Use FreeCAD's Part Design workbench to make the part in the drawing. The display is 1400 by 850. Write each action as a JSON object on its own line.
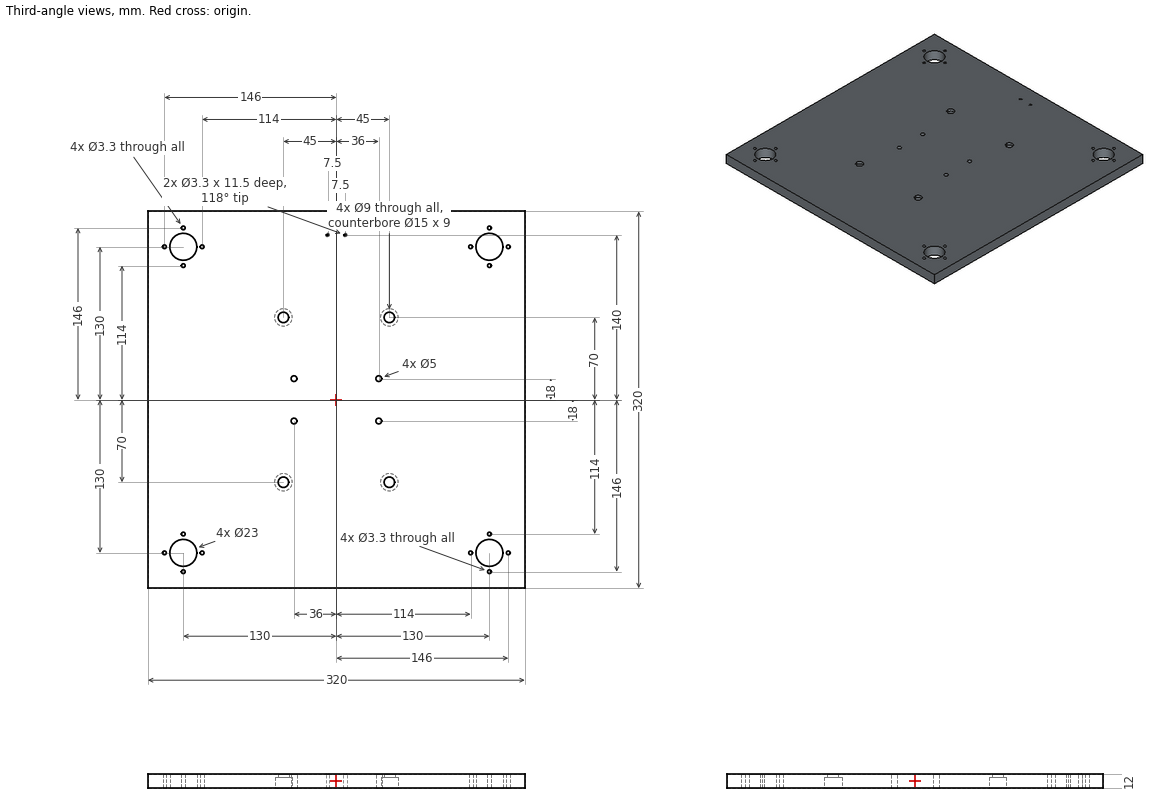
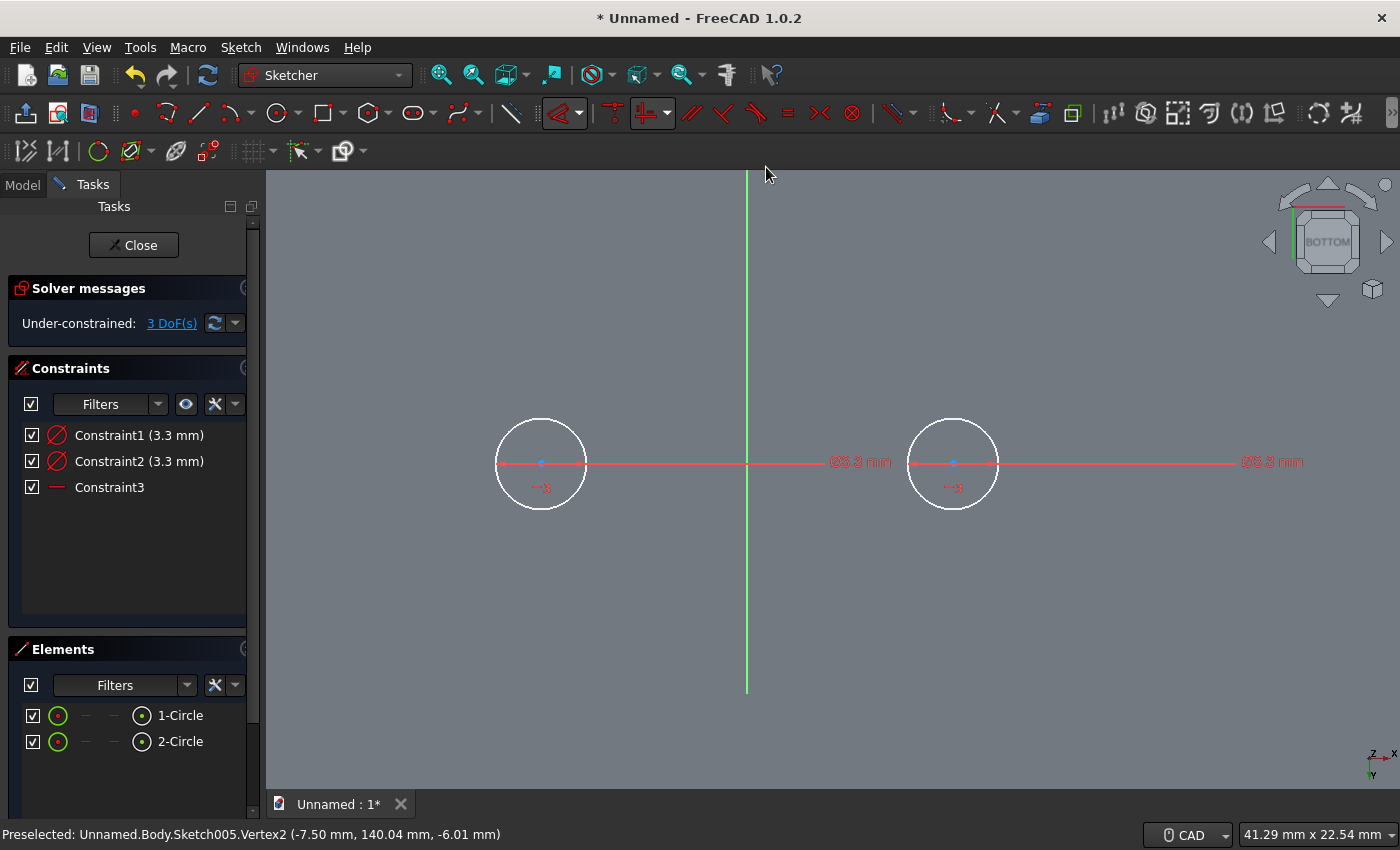
{"action": "left_click", "coordinate": [953, 464]}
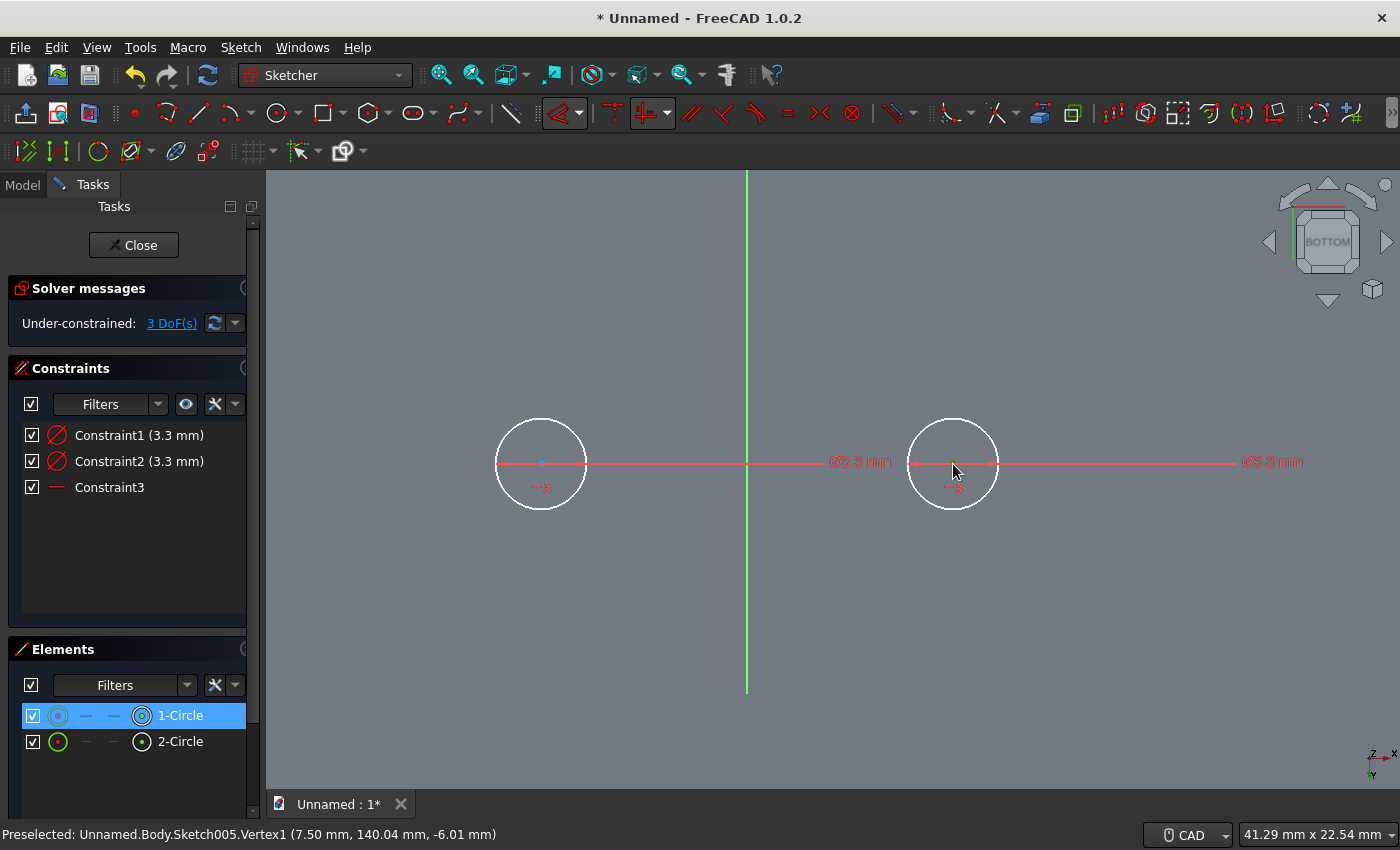
{"action": "key", "text": "l"}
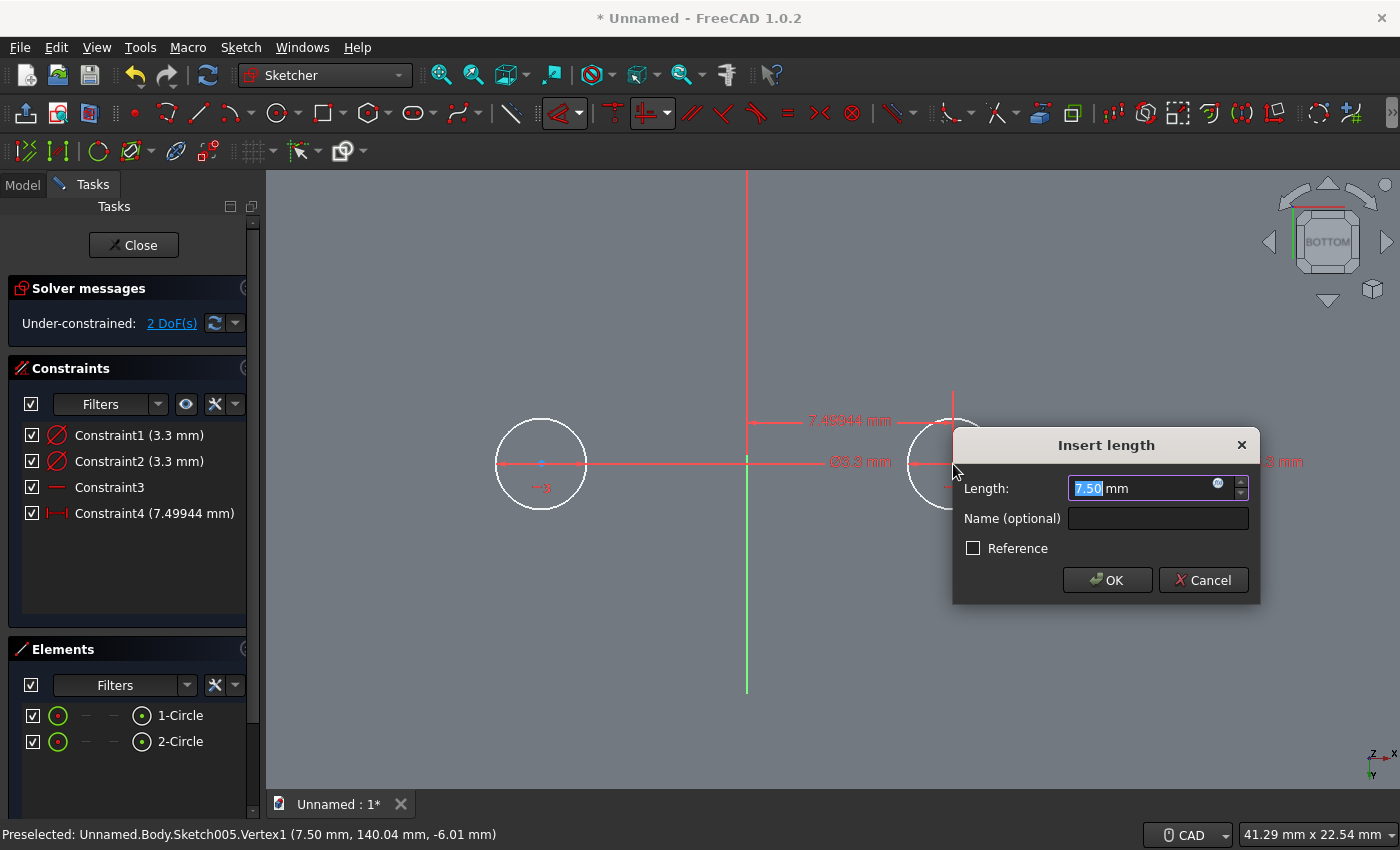
{"action": "type", "text": "7.5"}
{"action": "key", "text": "Return"}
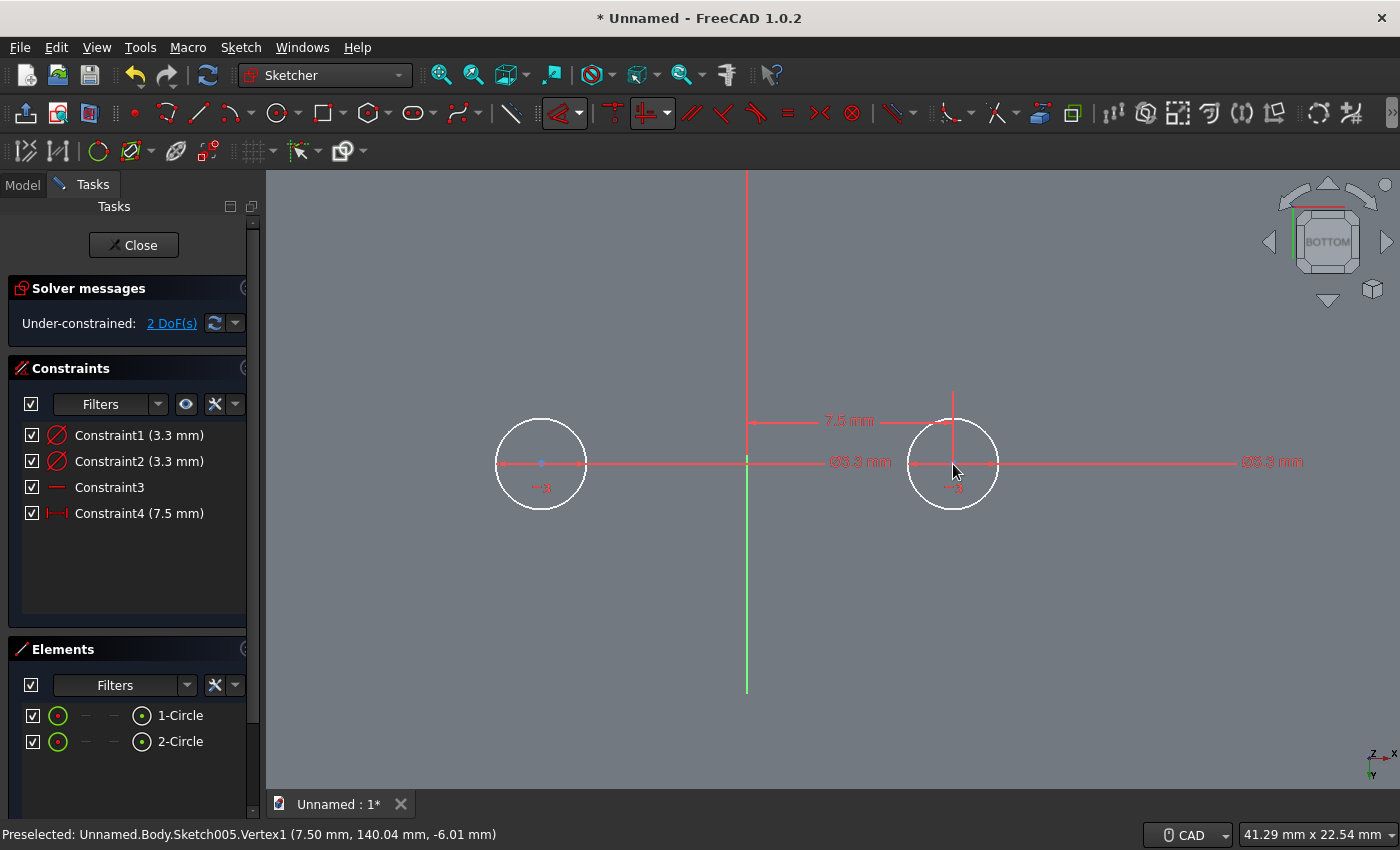
{"action": "left_click", "coordinate": [953, 464]}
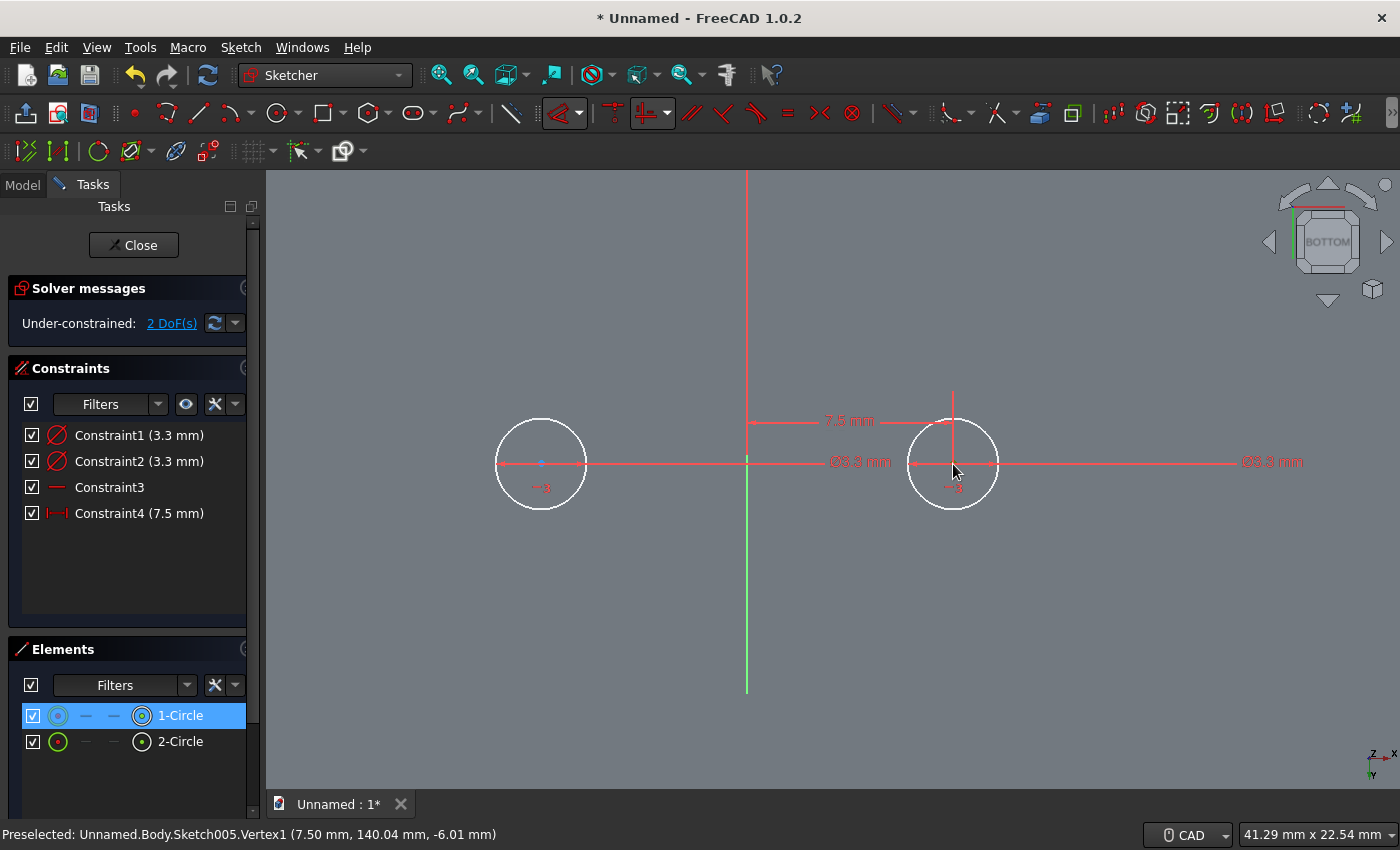
{"action": "left_click", "coordinate": [582, 114]}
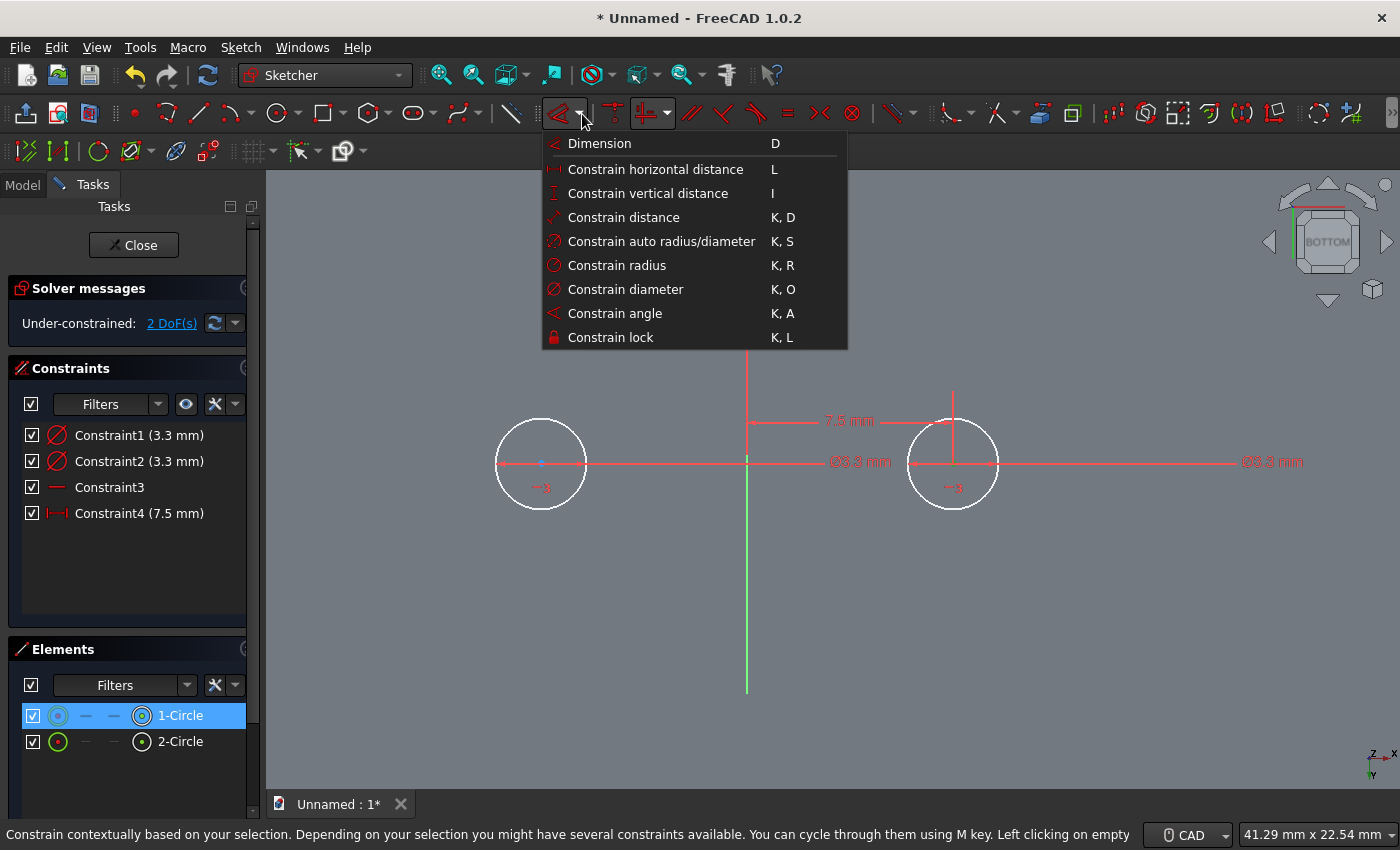
{"action": "left_click", "coordinate": [695, 193]}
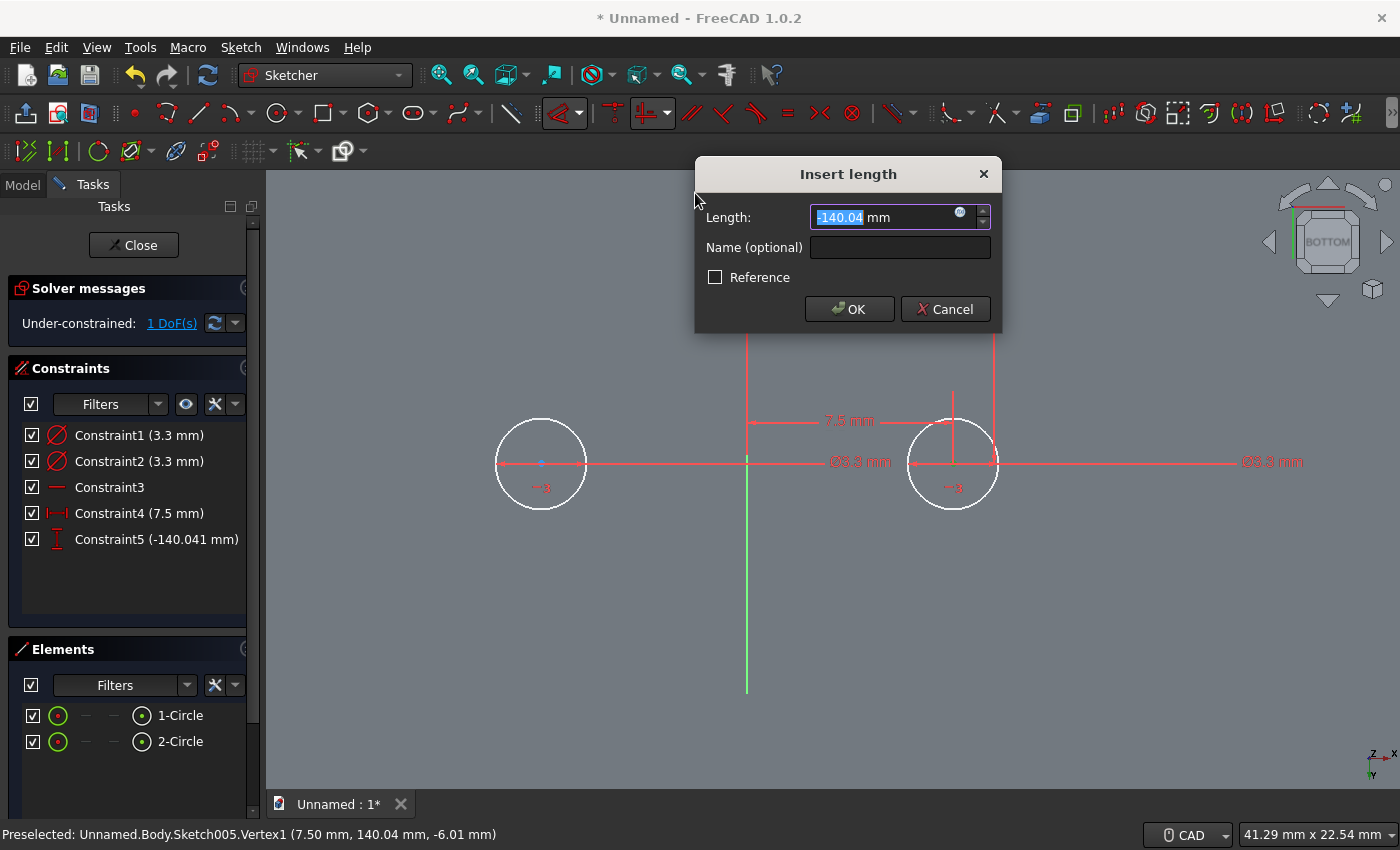
{"action": "type", "text": "-140"}
{"action": "key", "text": "Return"}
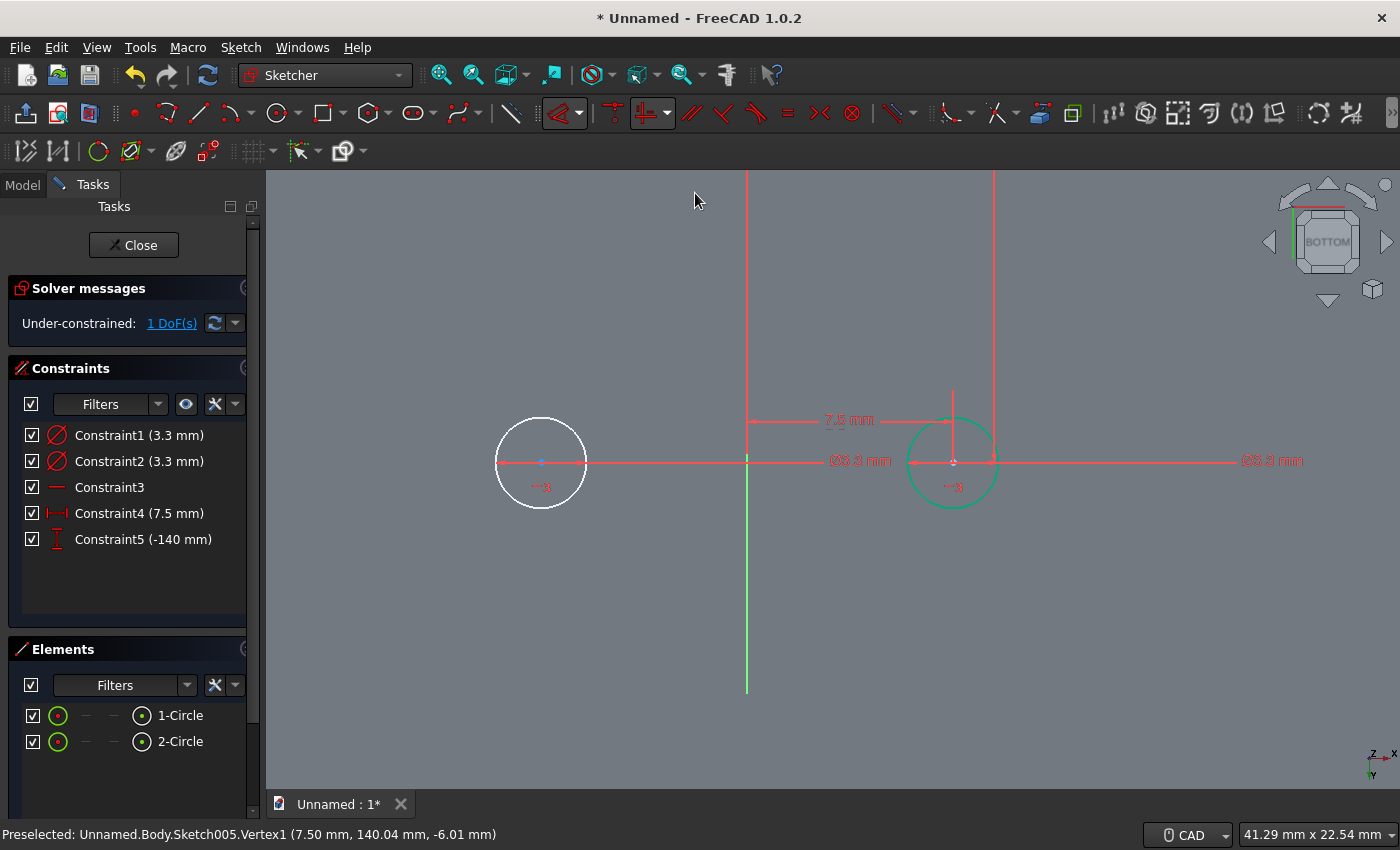
{"action": "left_click", "coordinate": [541, 463]}